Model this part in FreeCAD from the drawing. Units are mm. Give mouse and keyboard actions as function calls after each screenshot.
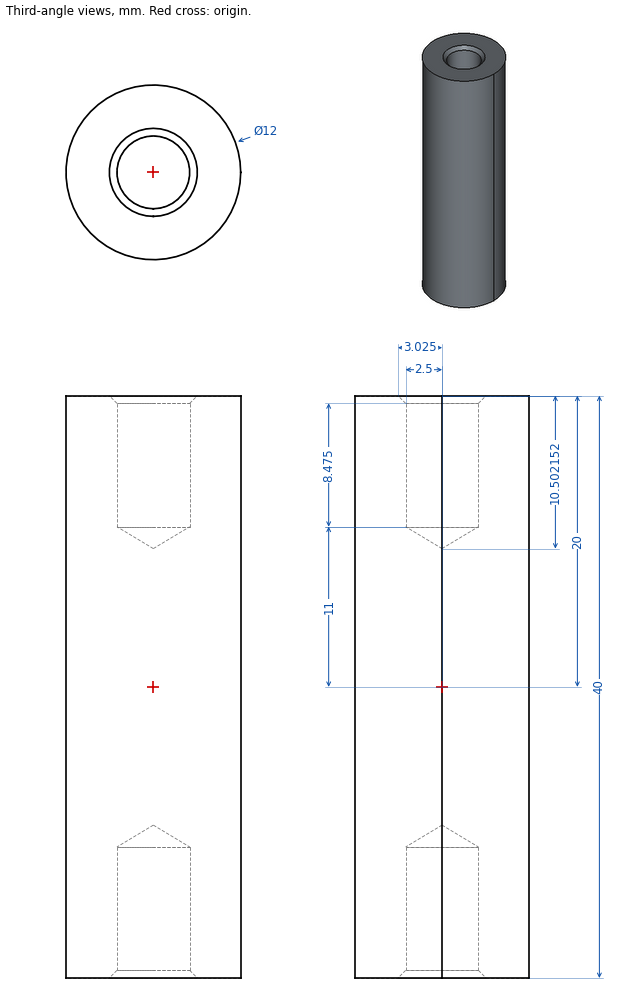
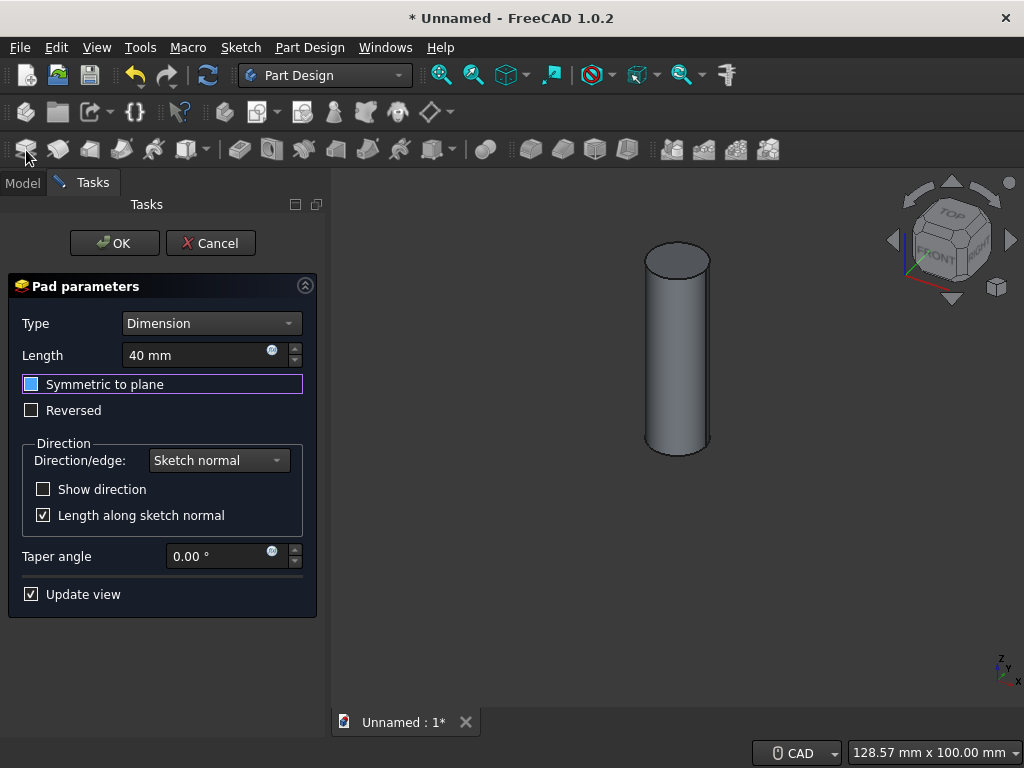
click(30, 384)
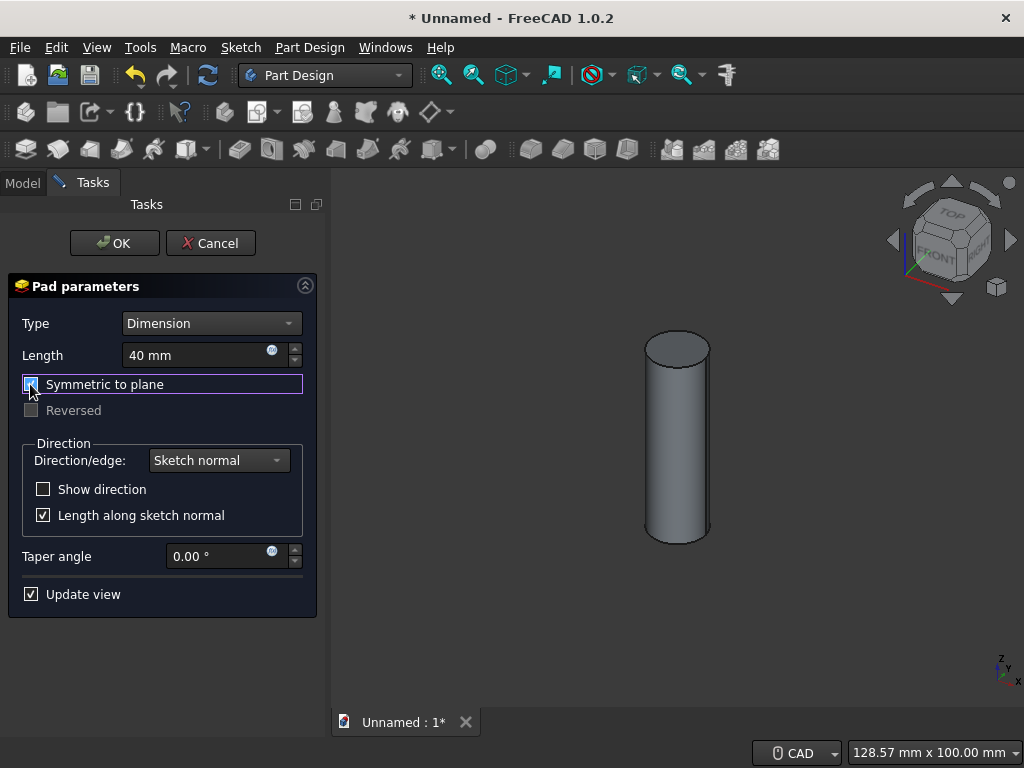
click(115, 243)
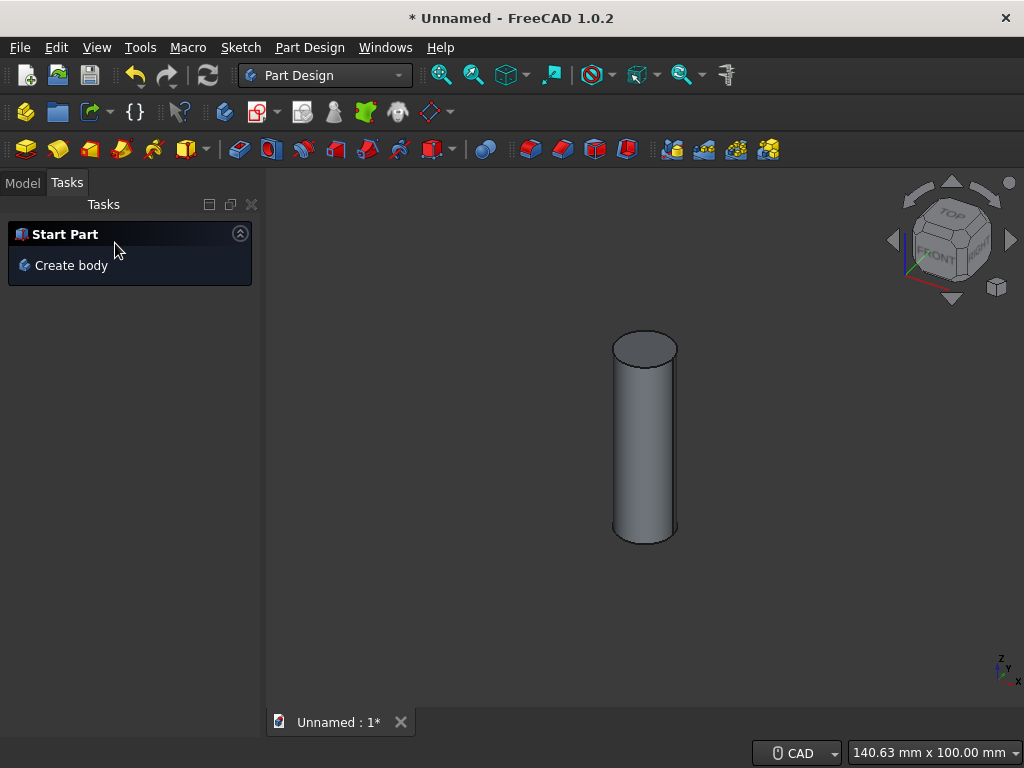
click(442, 76)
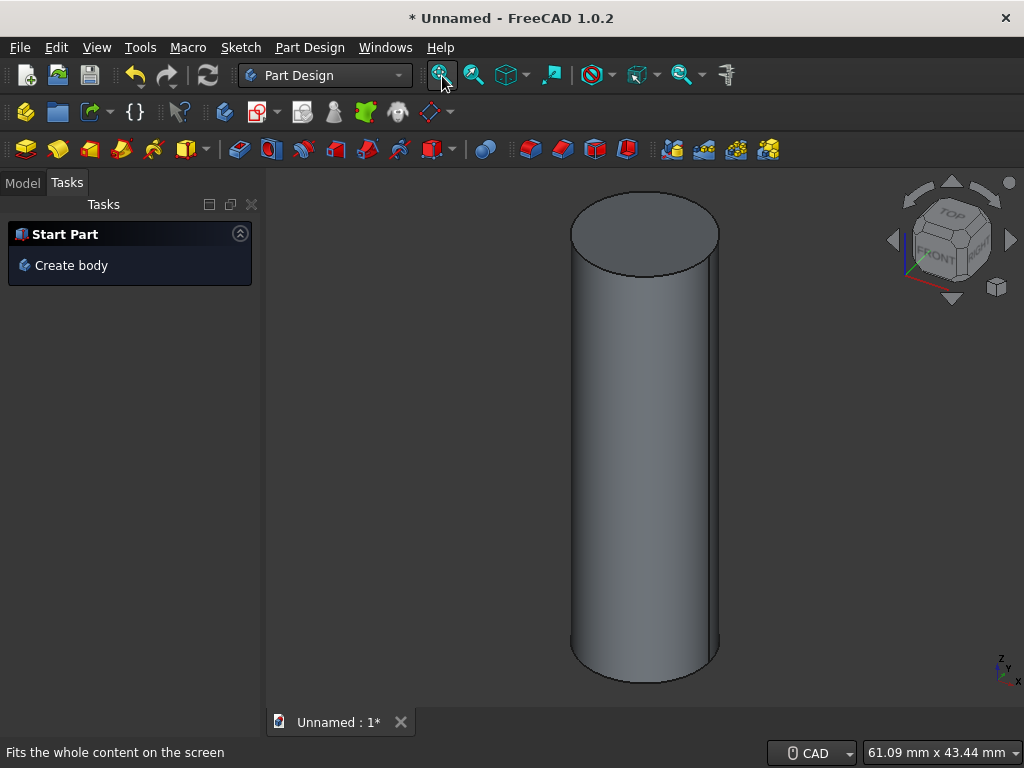
click(258, 112)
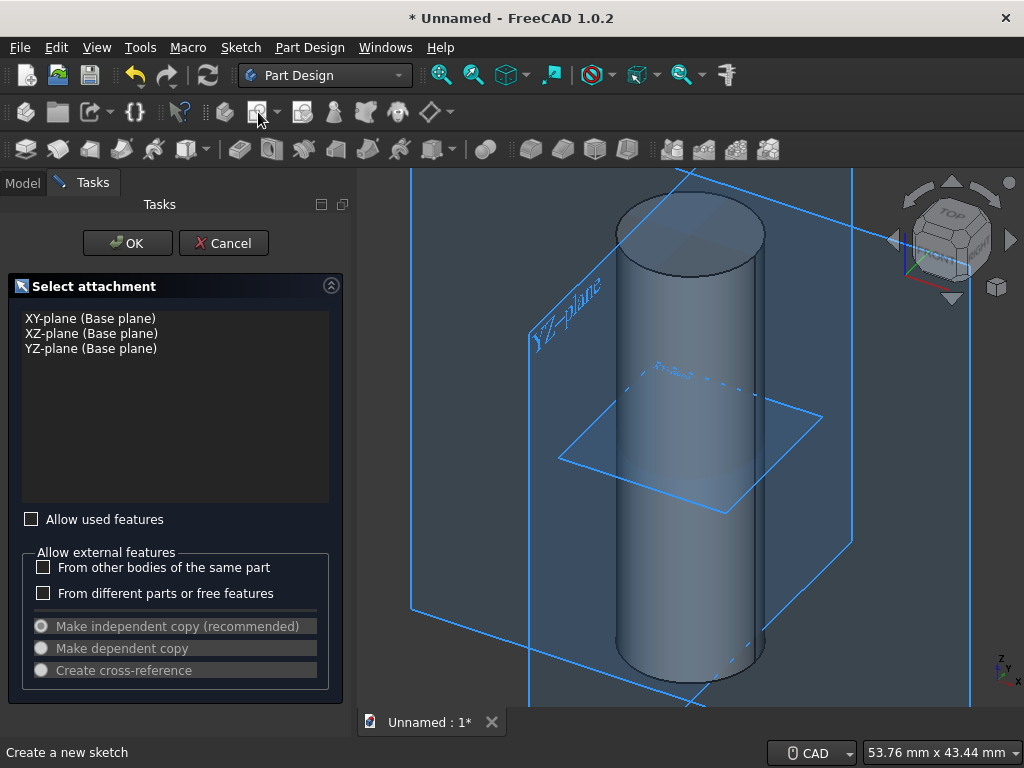
click(82, 348)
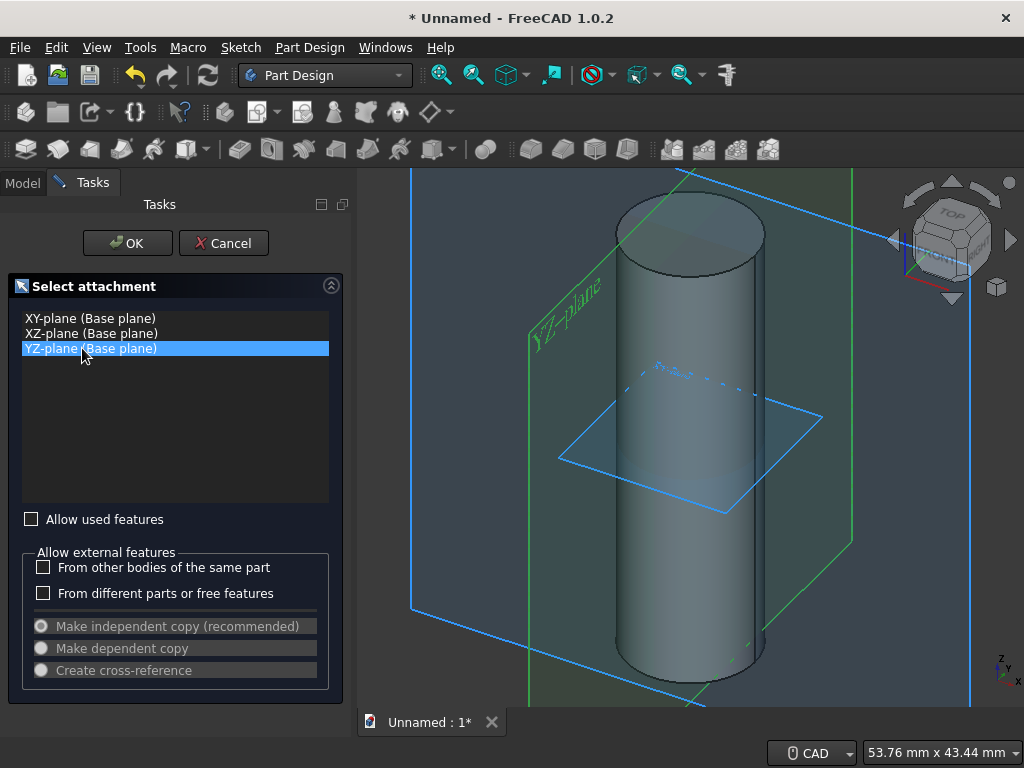
click(128, 243)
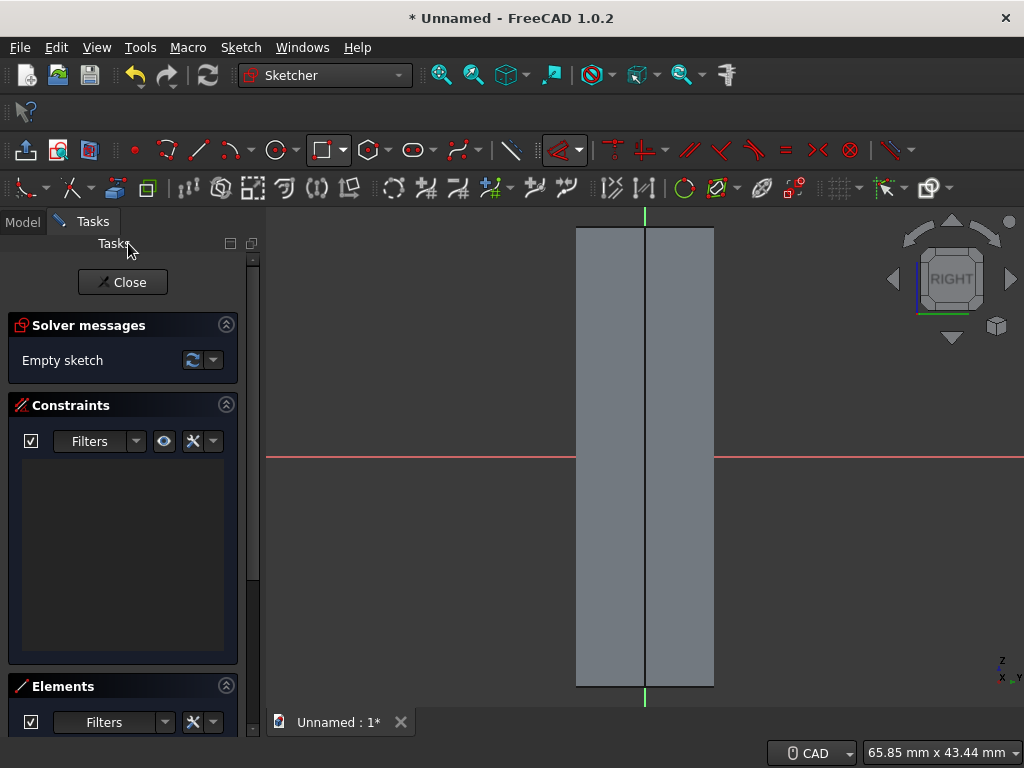
click(90, 150)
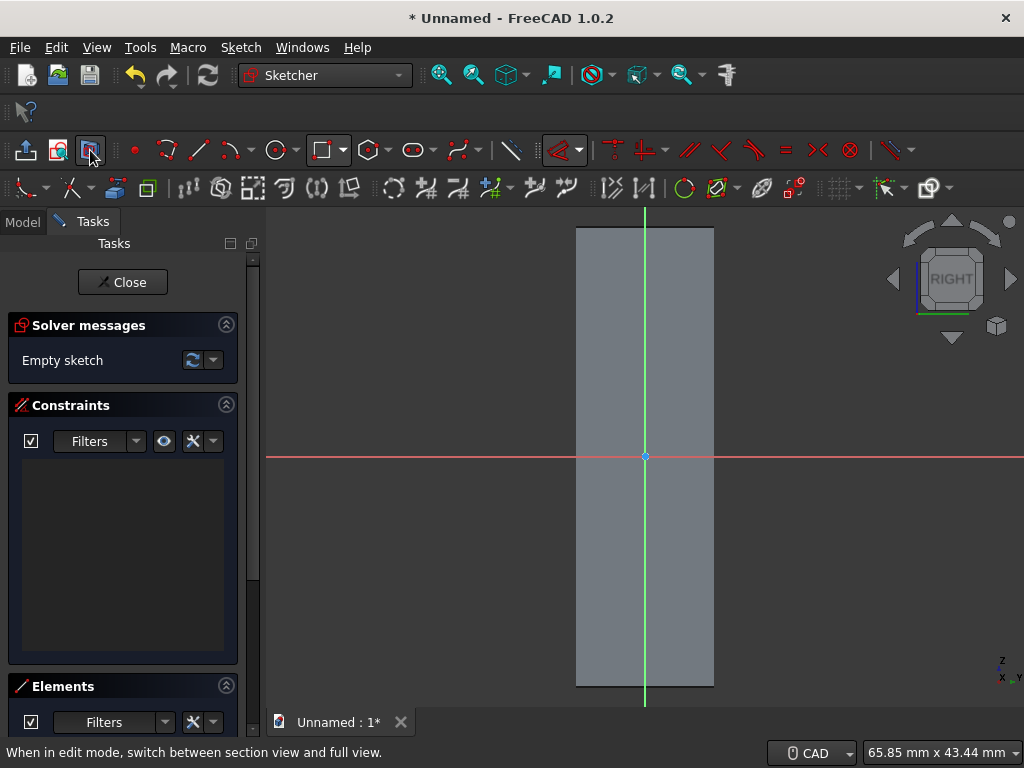
scroll(346, 679, down, 1)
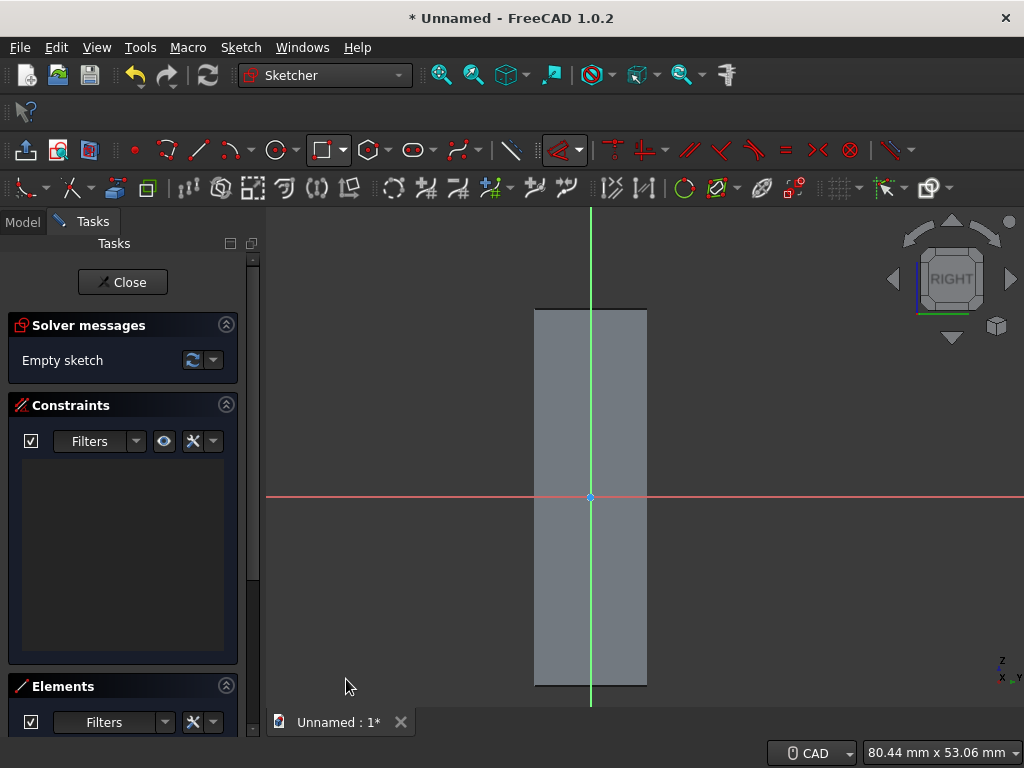
scroll(577, 338, up, 3)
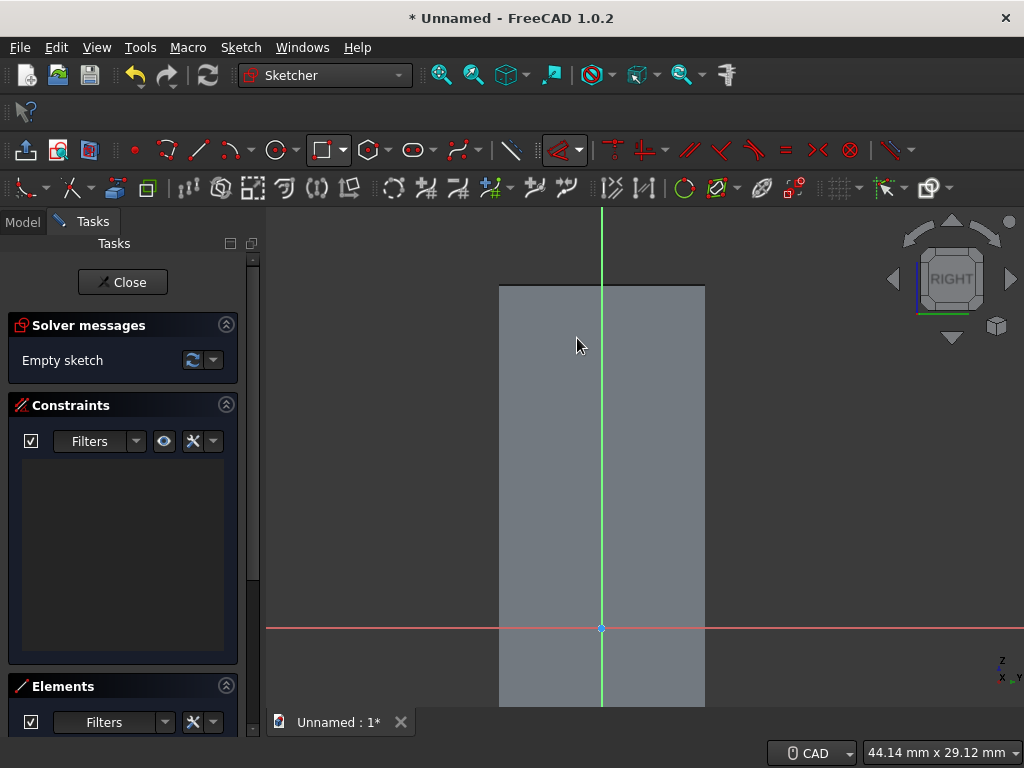
click(168, 150)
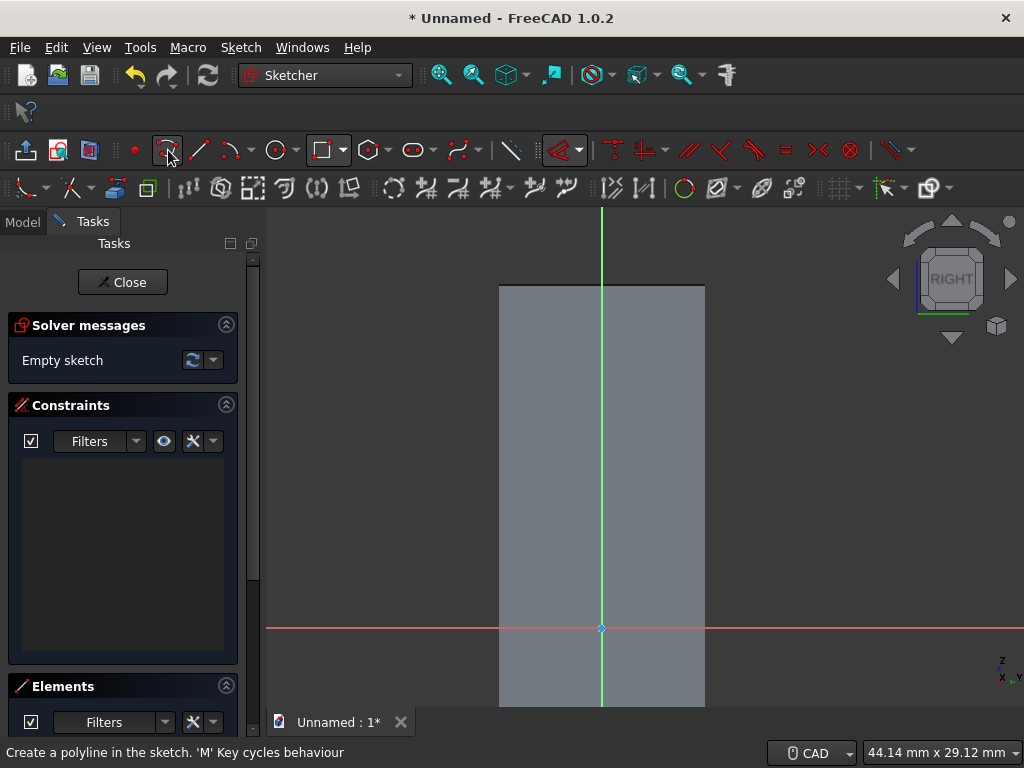
click(602, 465)
click(593, 285)
click(550, 285)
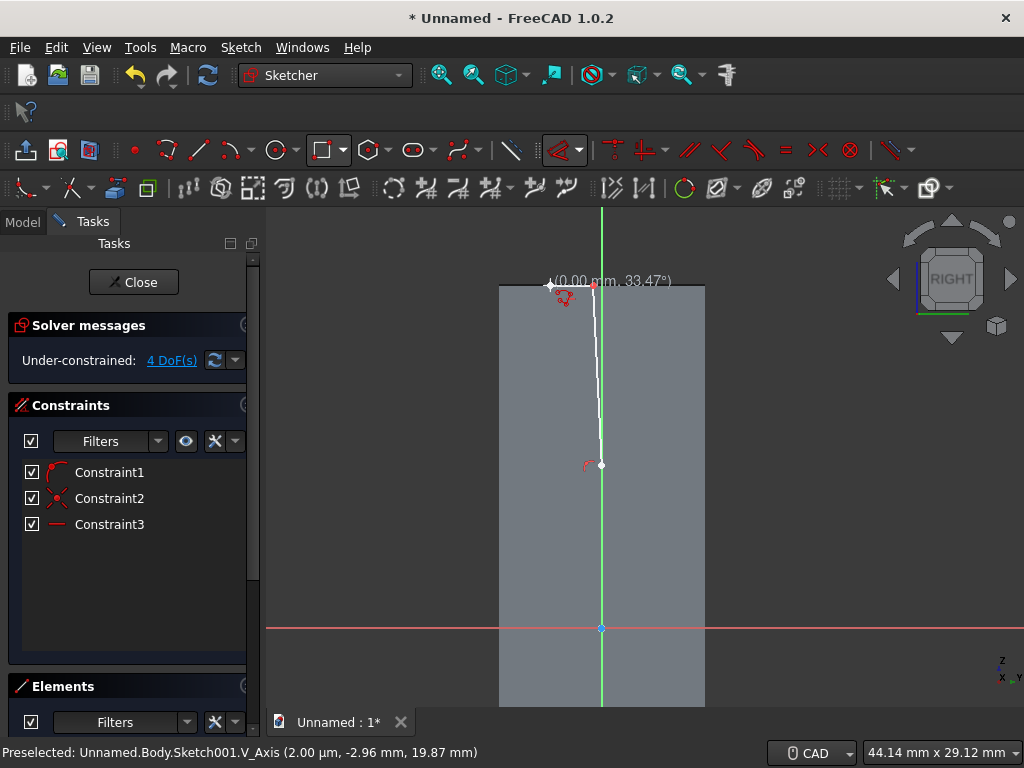
scroll(559, 294, up, 3)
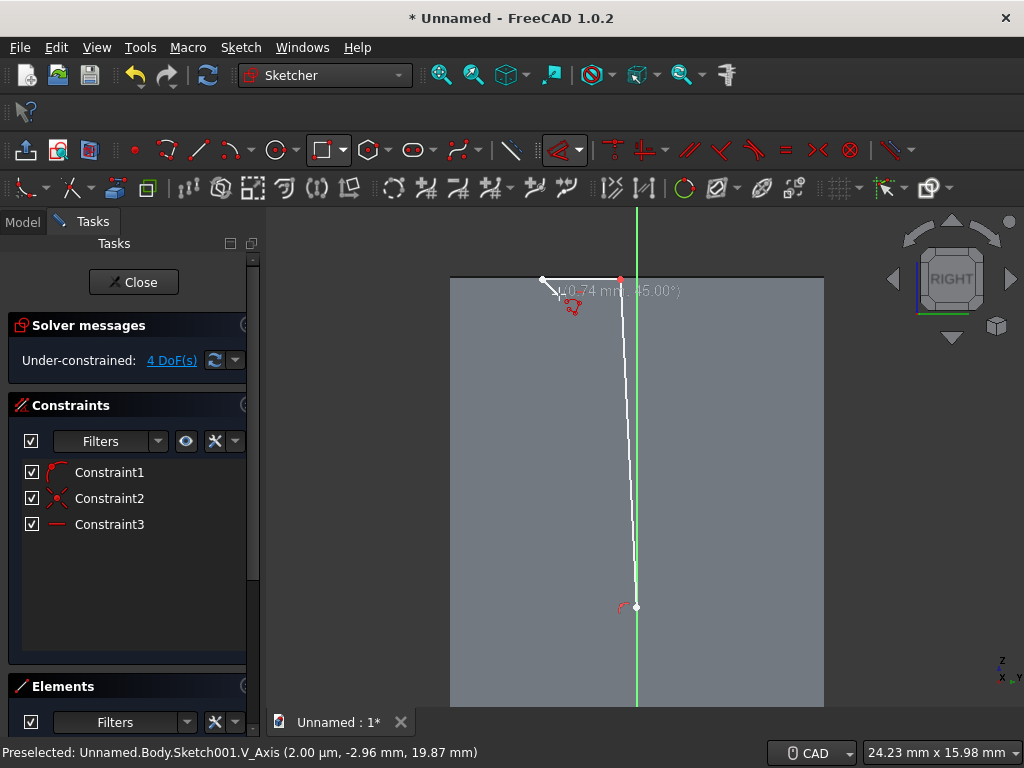
click(559, 294)
click(559, 559)
click(637, 607)
key(Escape)
key(Escape)